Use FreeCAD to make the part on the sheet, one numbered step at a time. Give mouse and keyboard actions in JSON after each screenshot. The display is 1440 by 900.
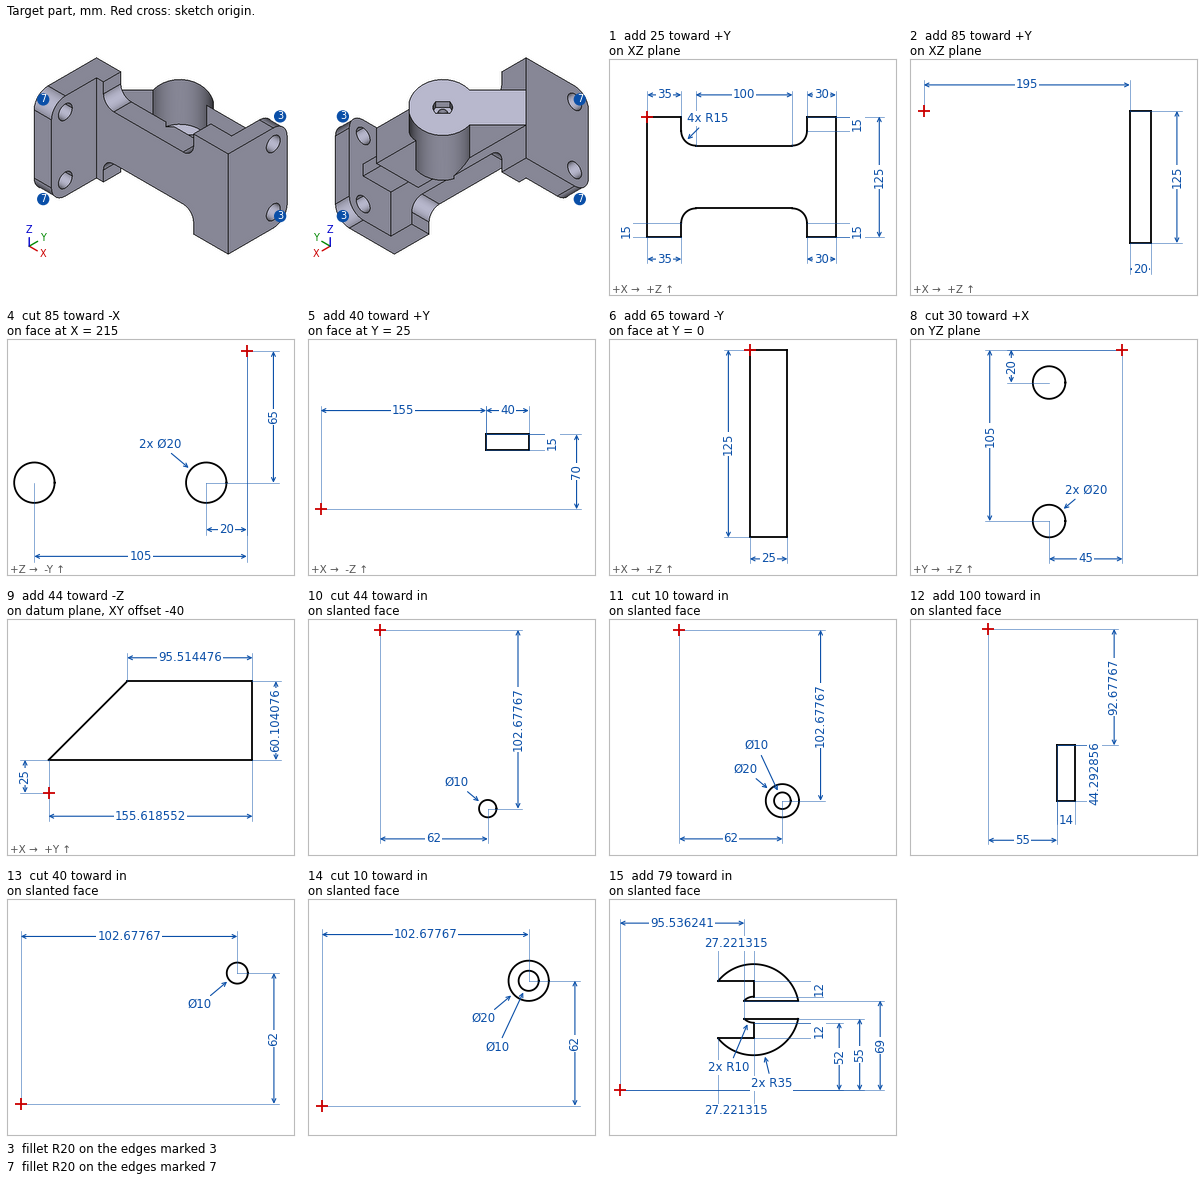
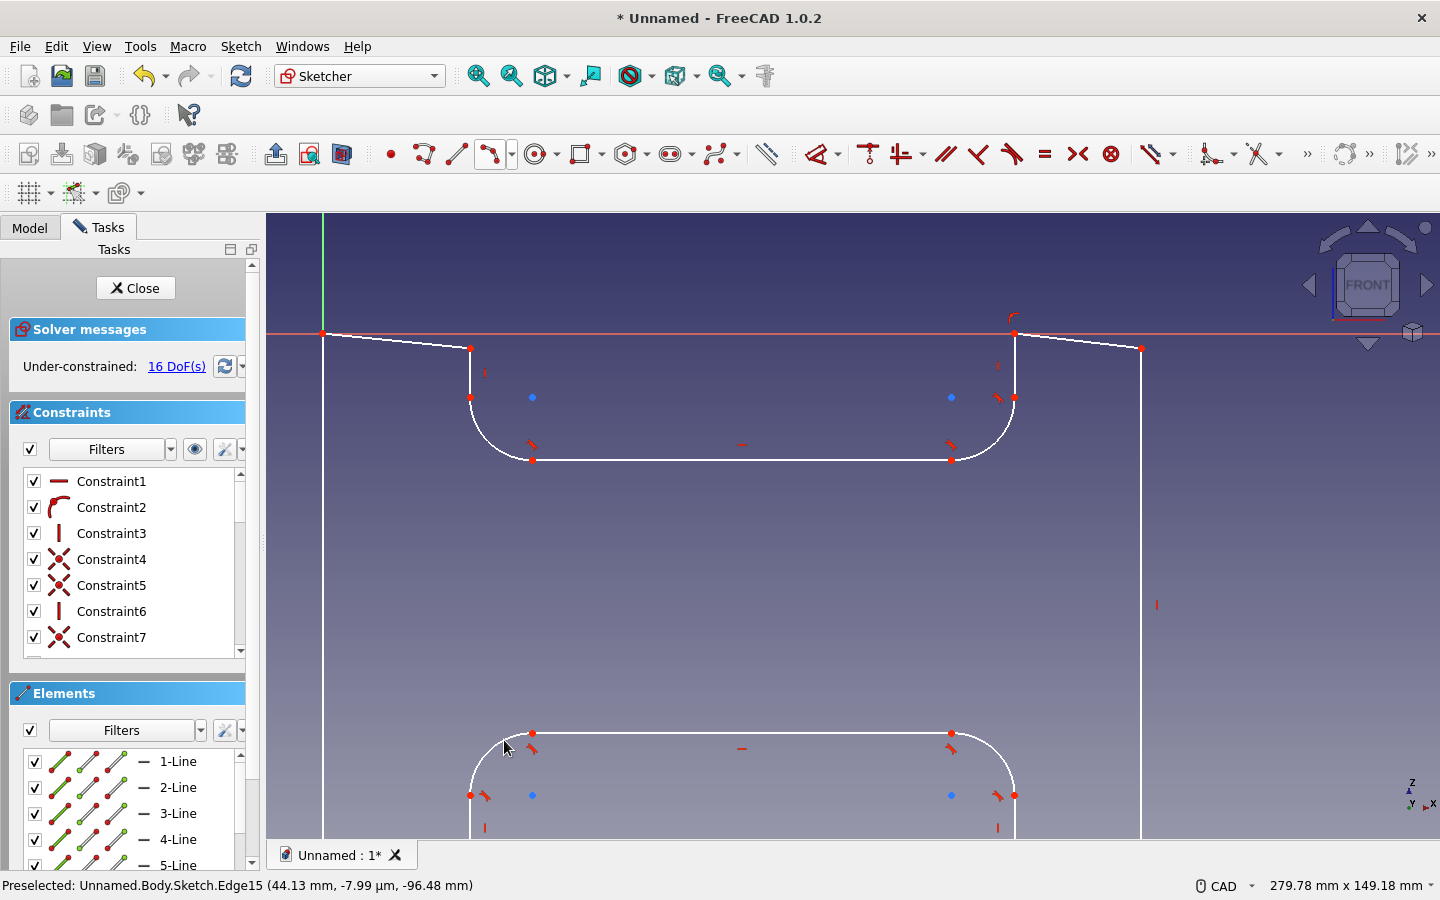
{"action": "left_click", "coordinate": [470, 363]}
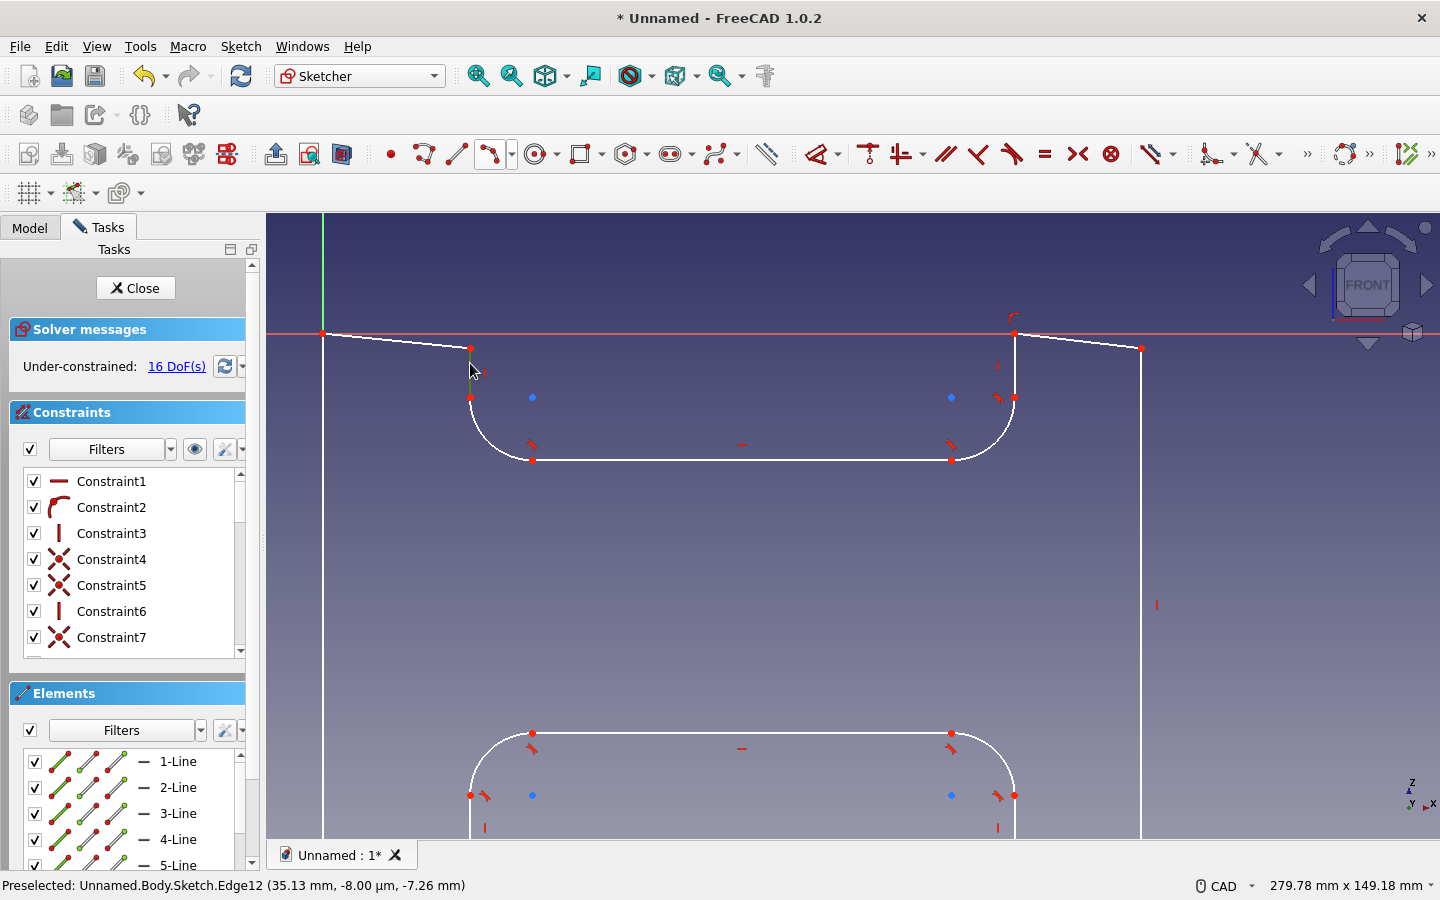
{"action": "left_click", "coordinate": [477, 426]}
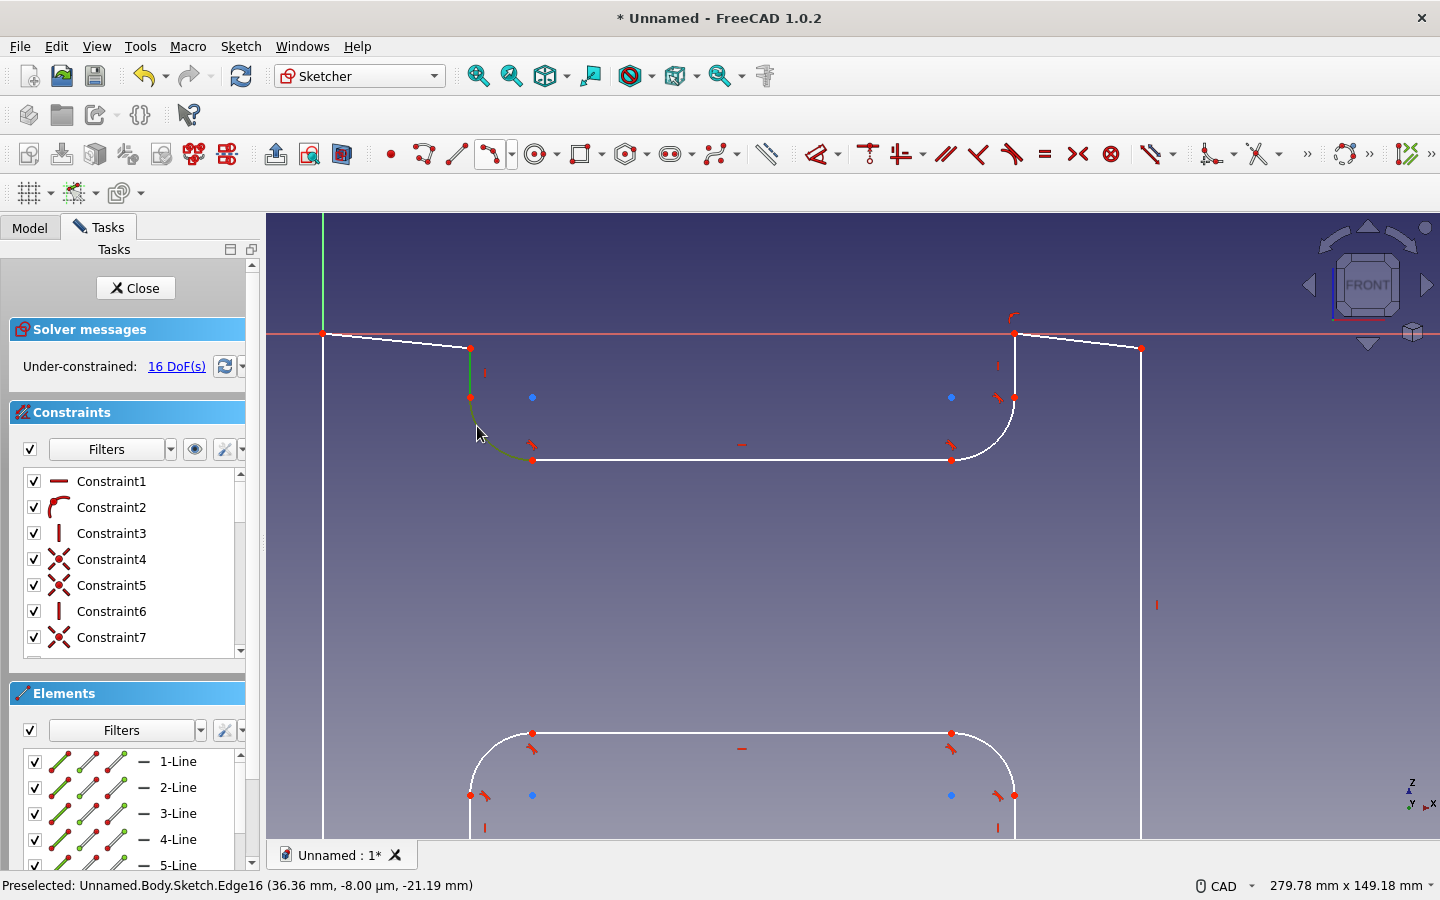
{"action": "left_click", "coordinate": [1012, 154]}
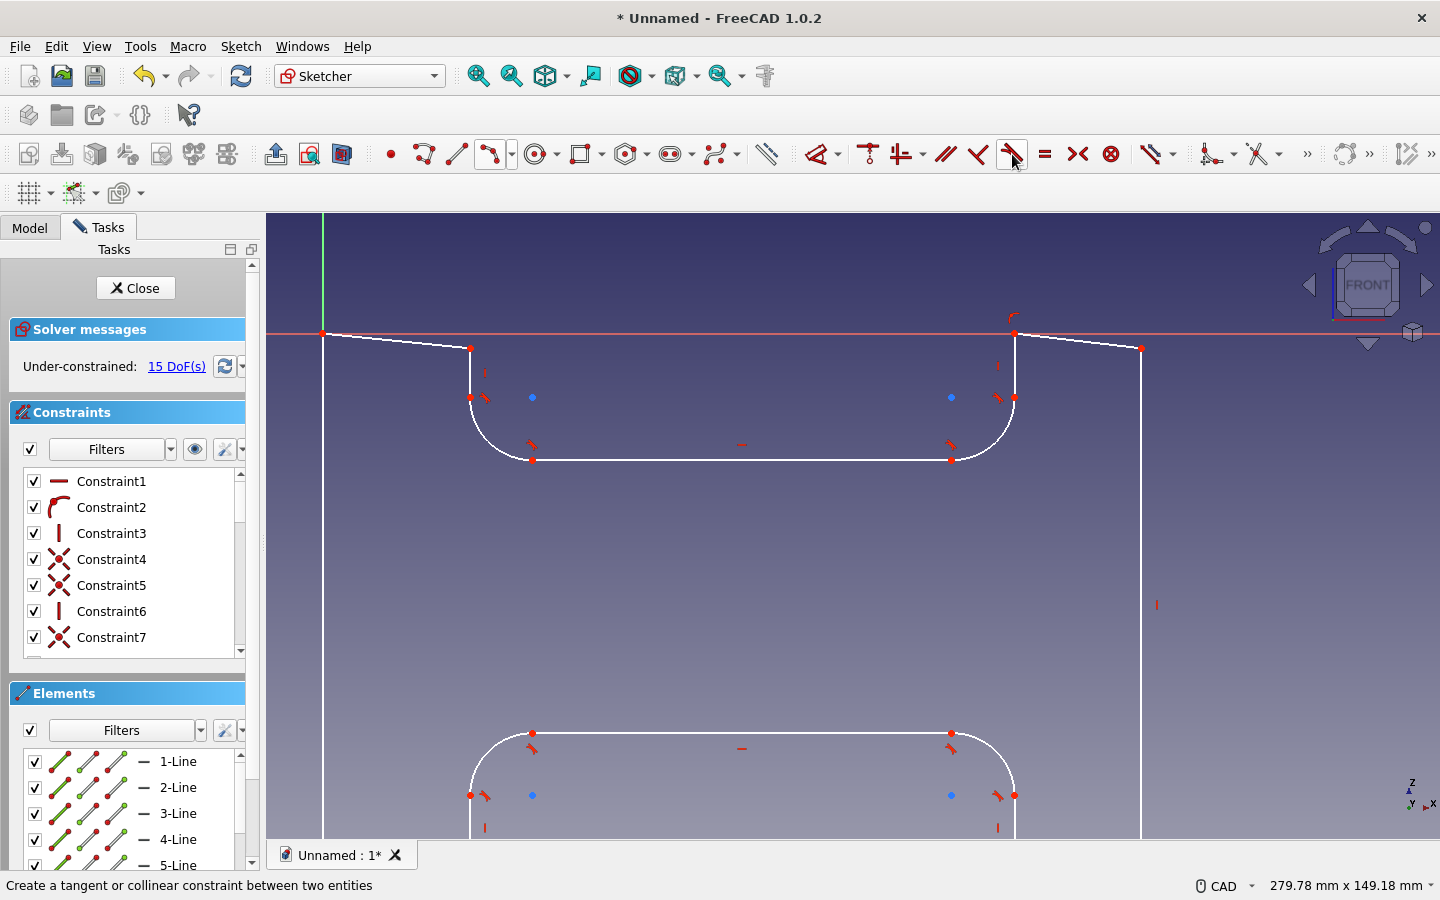
{"action": "scroll", "coordinate": [1103, 344], "scroll_direction": "up", "scroll_amount": 2}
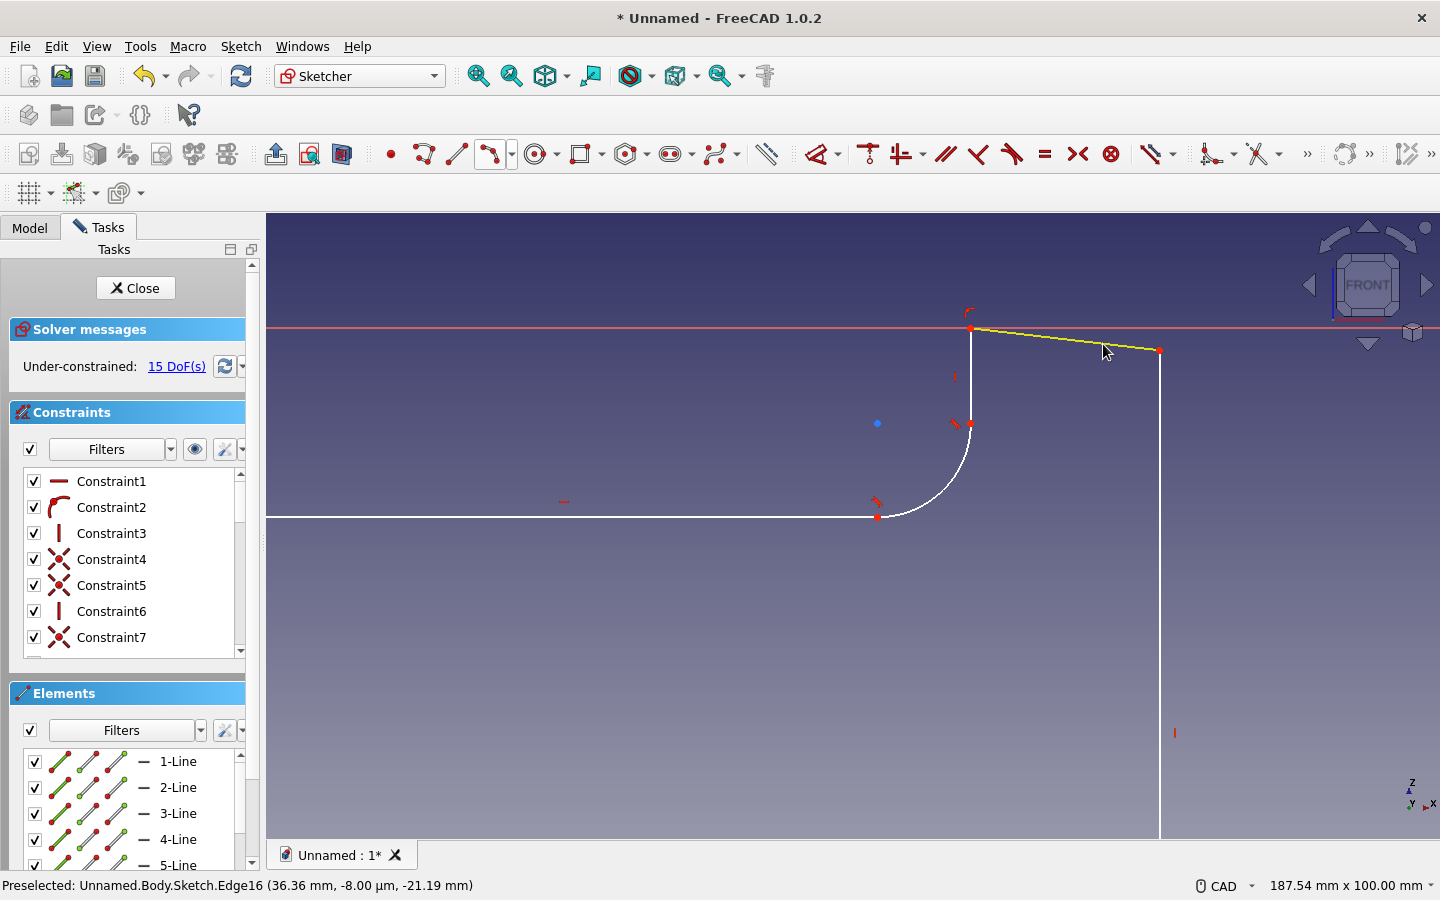
{"action": "left_click", "coordinate": [1103, 344]}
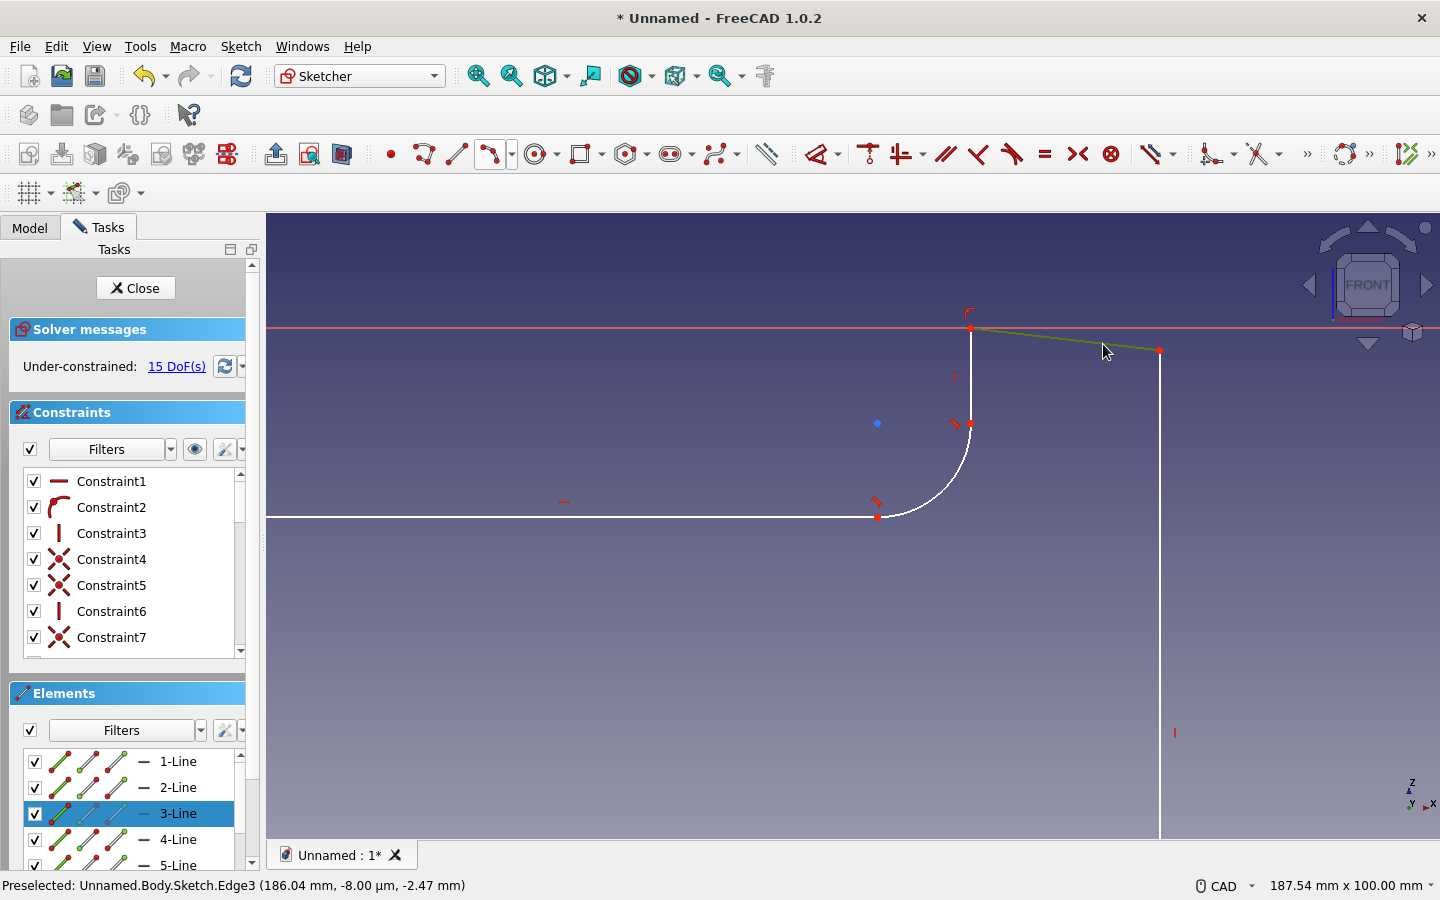
{"action": "key", "text": "h"}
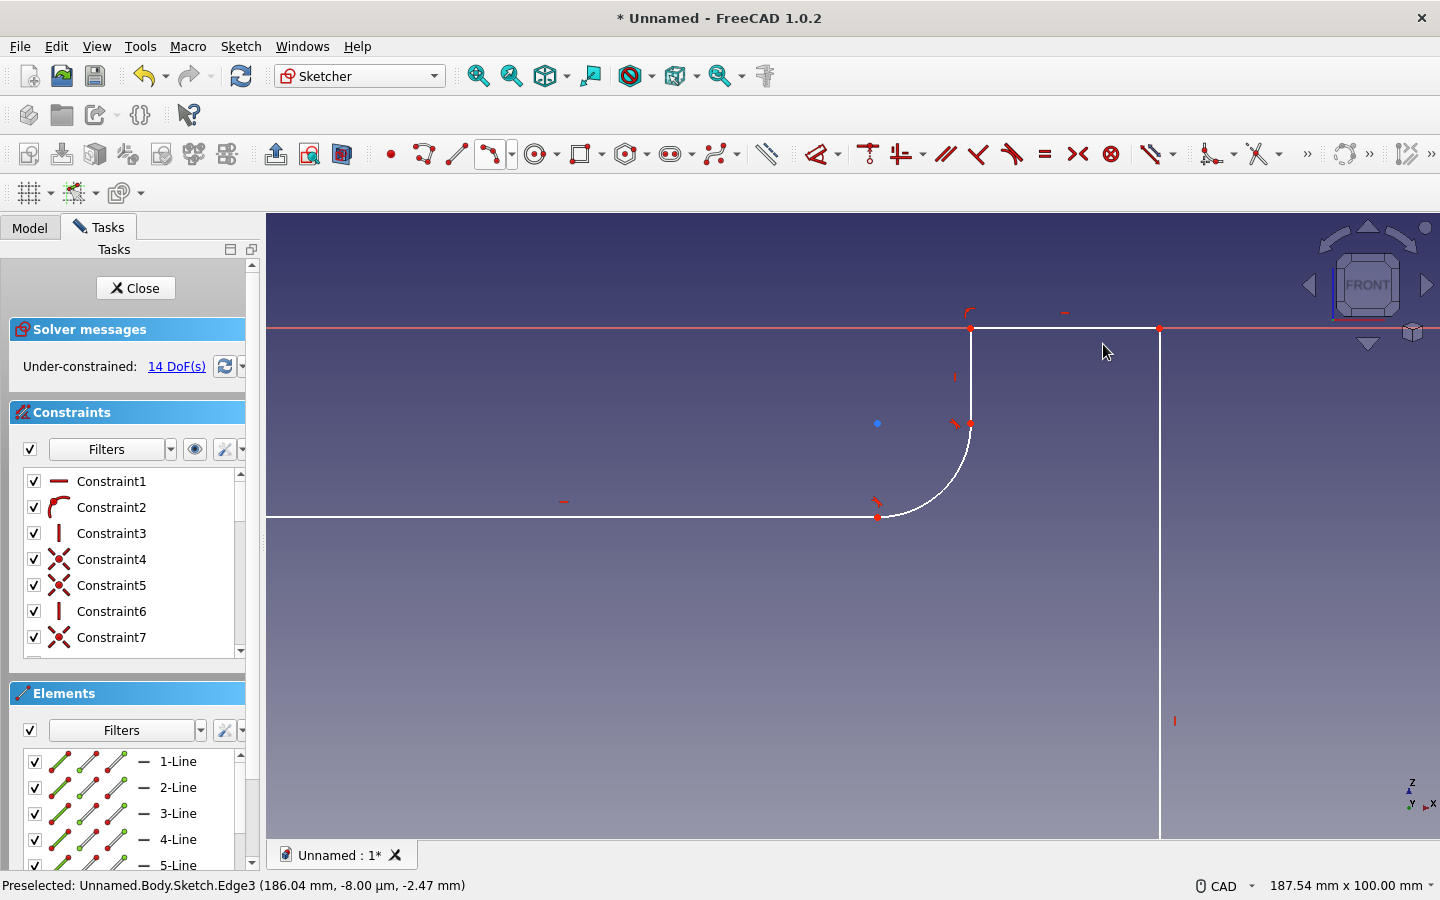
{"action": "scroll", "coordinate": [1071, 291], "scroll_direction": "down", "scroll_amount": 3}